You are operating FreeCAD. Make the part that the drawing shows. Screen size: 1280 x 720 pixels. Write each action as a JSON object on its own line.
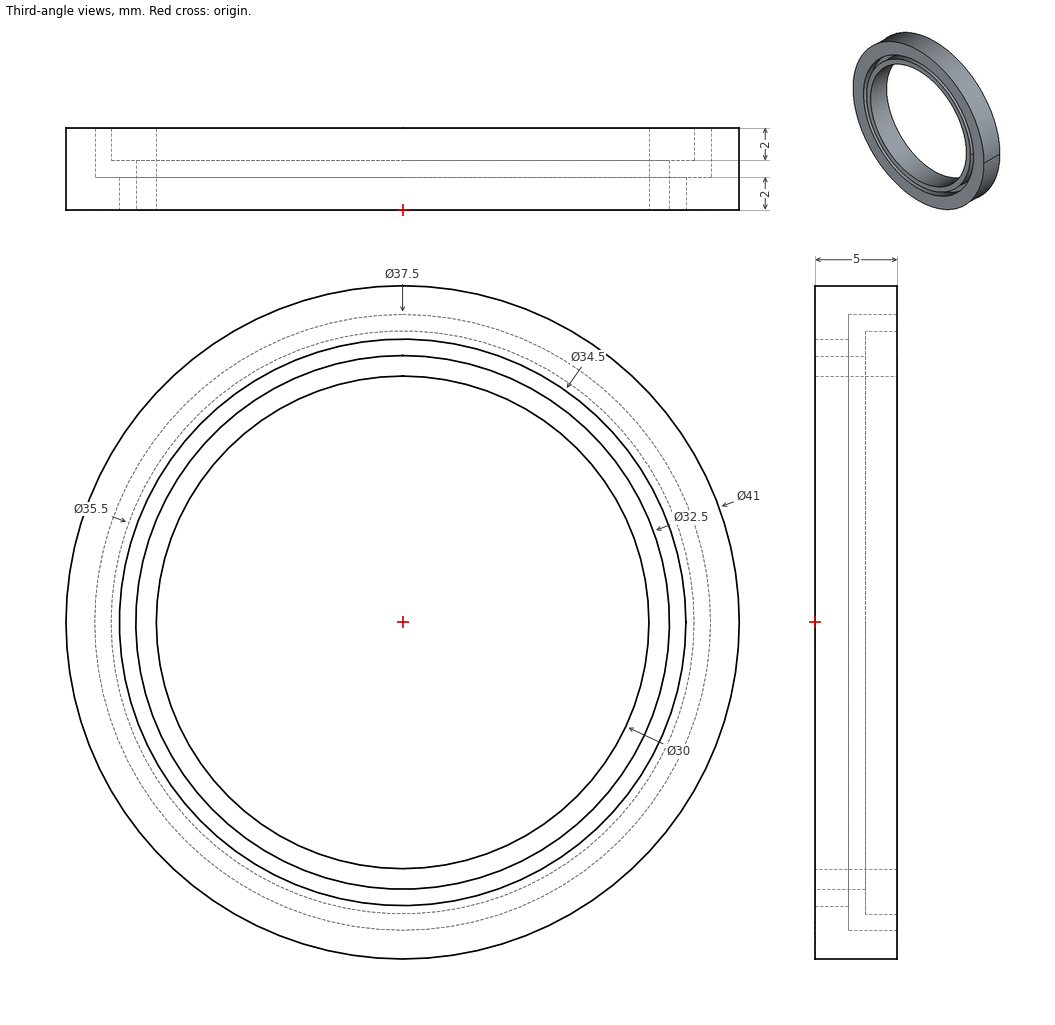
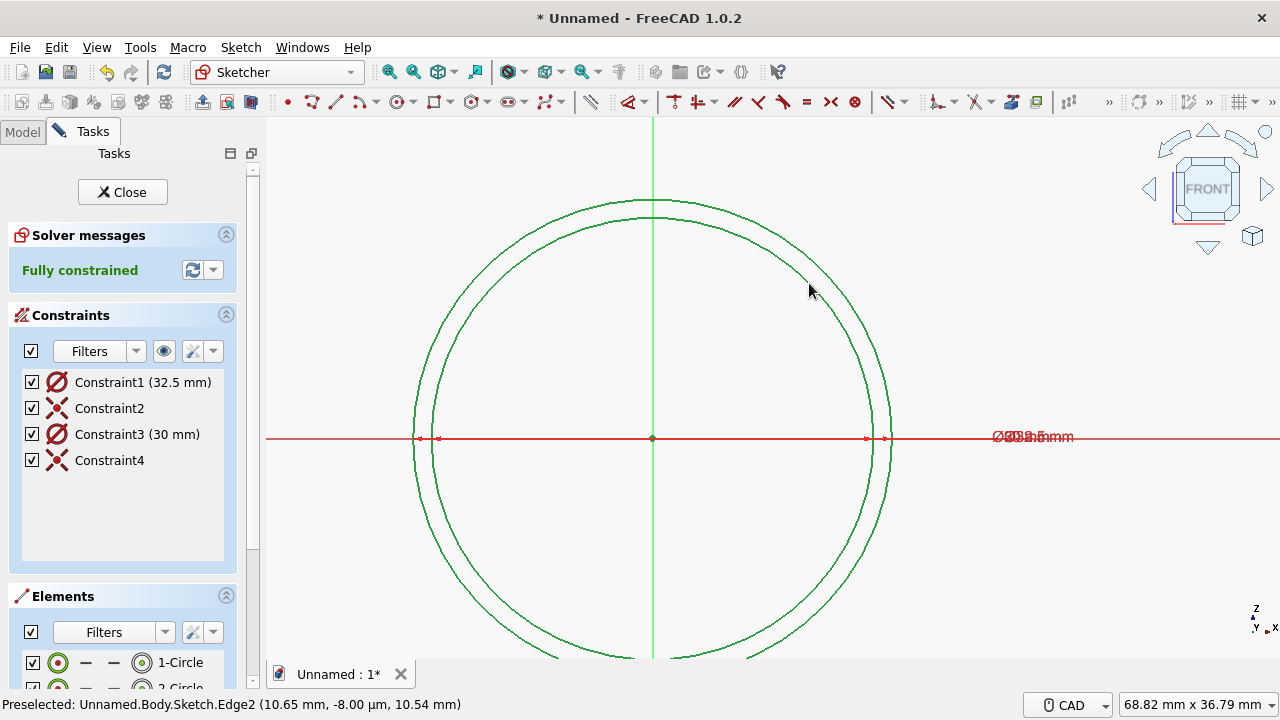
{"action": "left_click", "coordinate": [123, 192]}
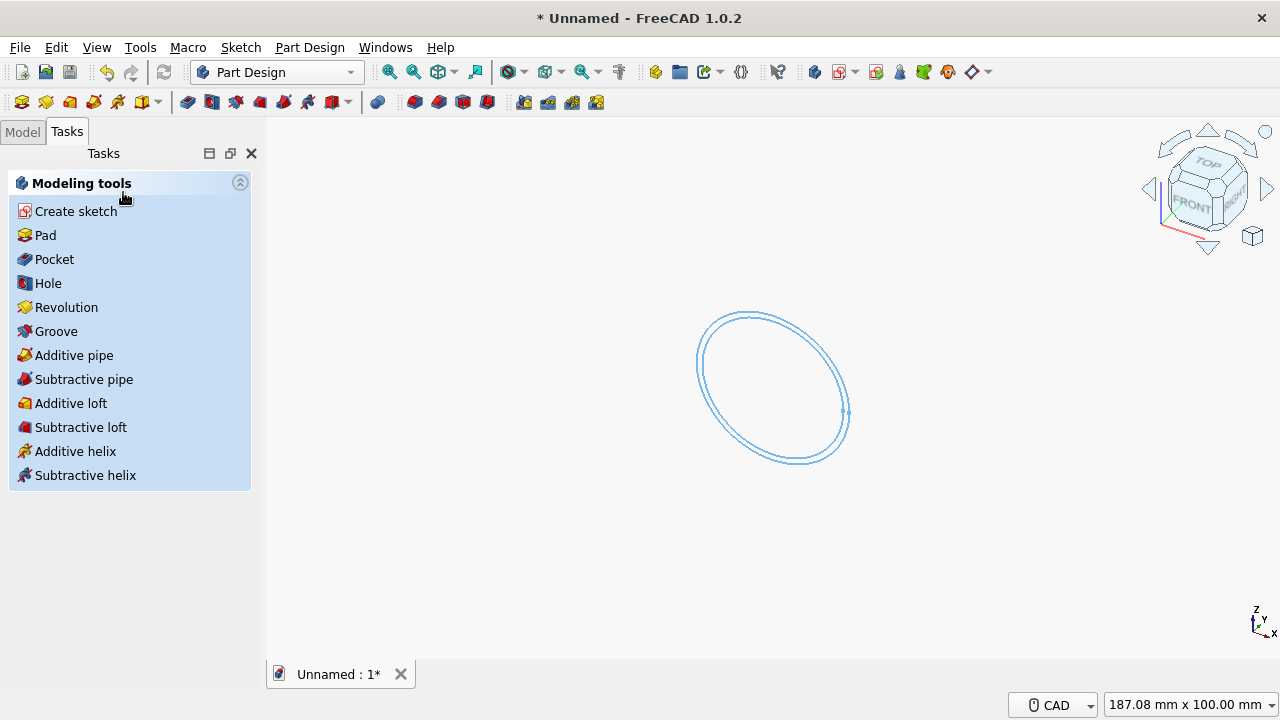
{"action": "left_click", "coordinate": [22, 102]}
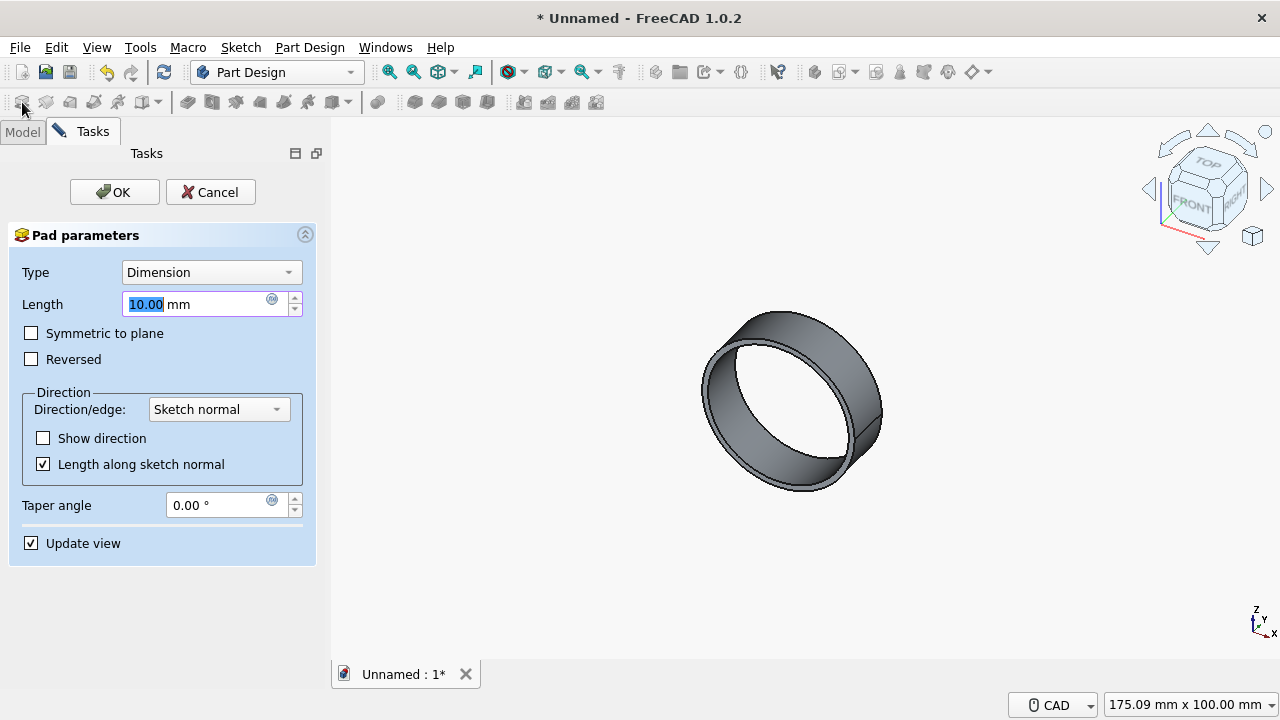
{"action": "type", "text": "5"}
{"action": "key", "text": "Tab"}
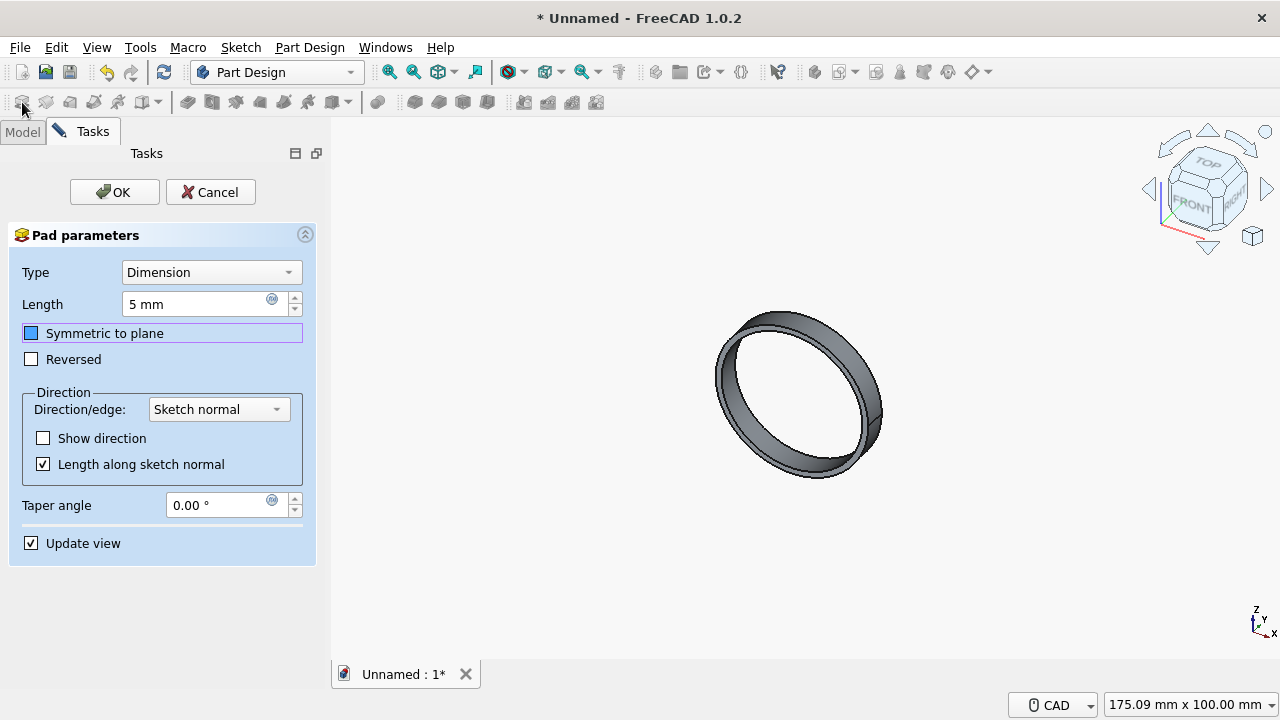
{"action": "left_click", "coordinate": [30, 359]}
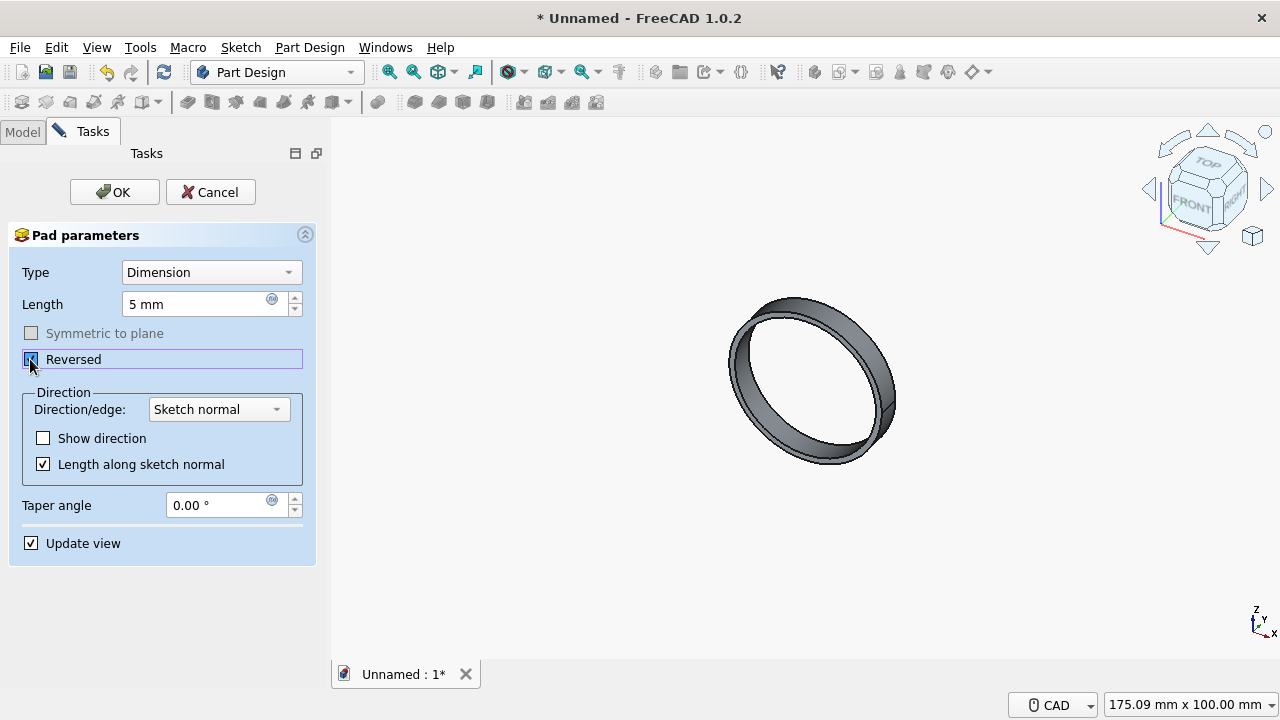
{"action": "left_click", "coordinate": [115, 192]}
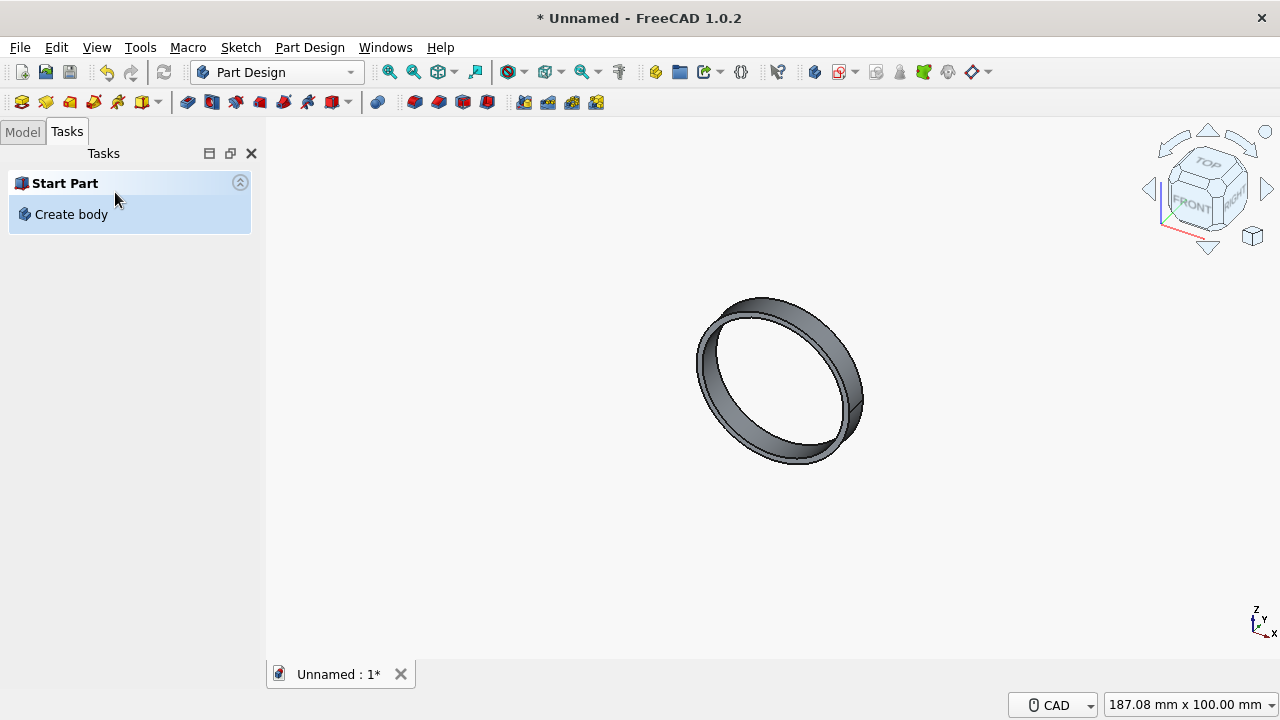
{"action": "key", "text": "v f"}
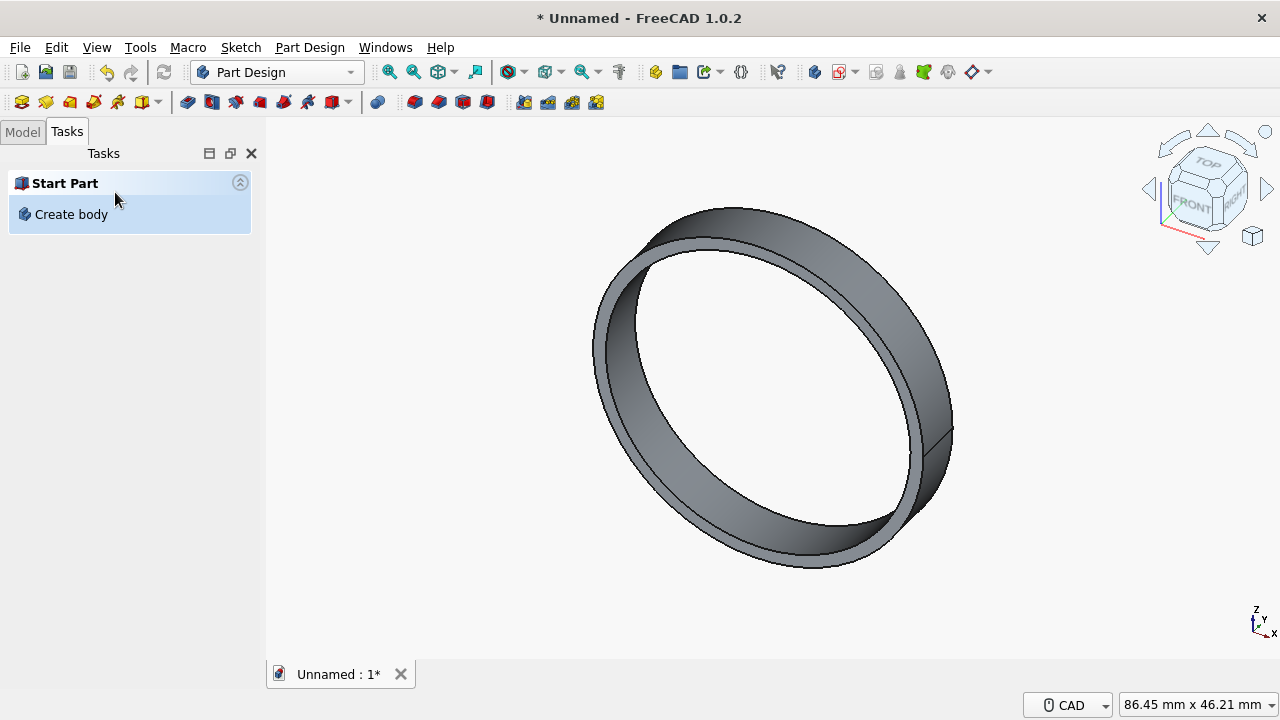
{"action": "left_click", "coordinate": [23, 131]}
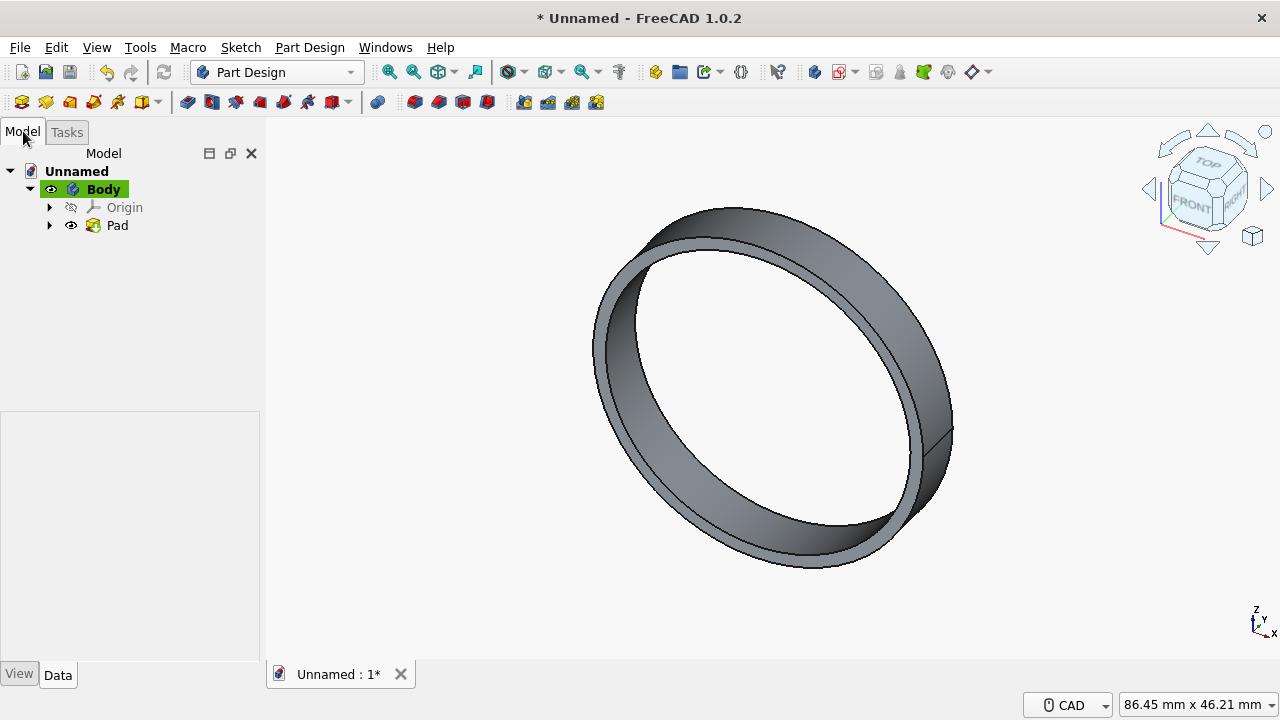
{"action": "left_click", "coordinate": [50, 207]}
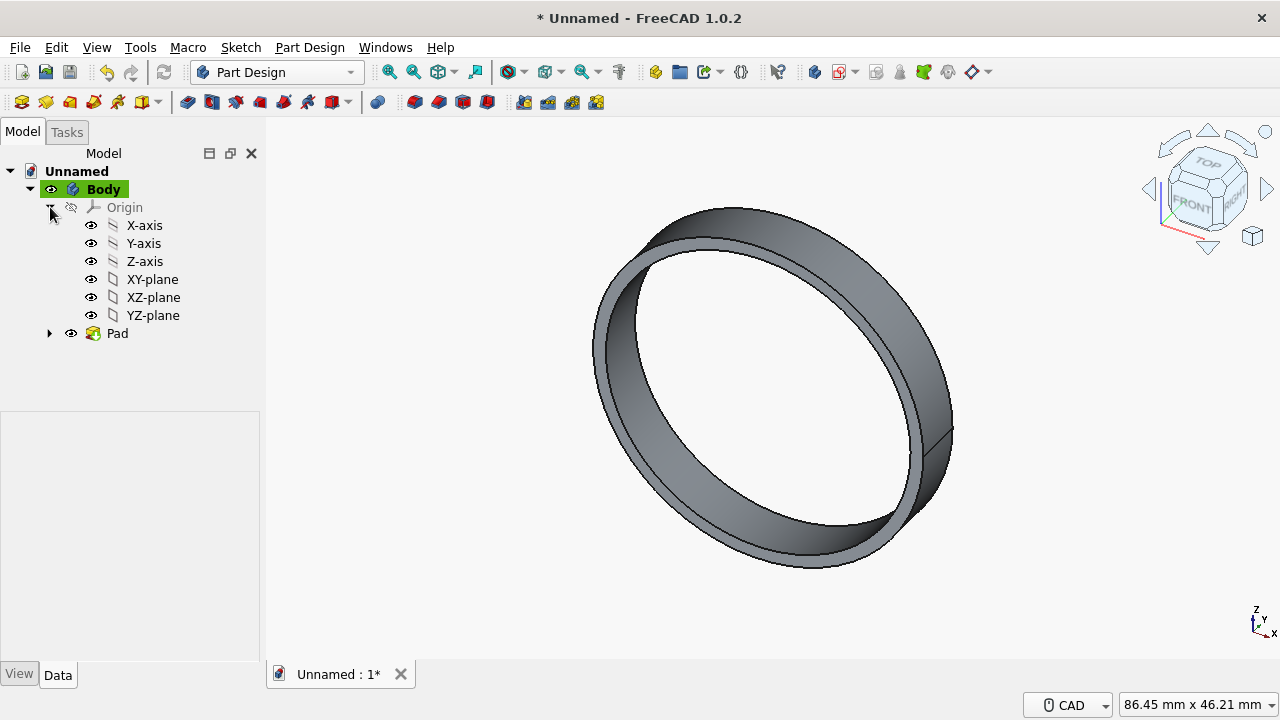
{"action": "left_click", "coordinate": [136, 297]}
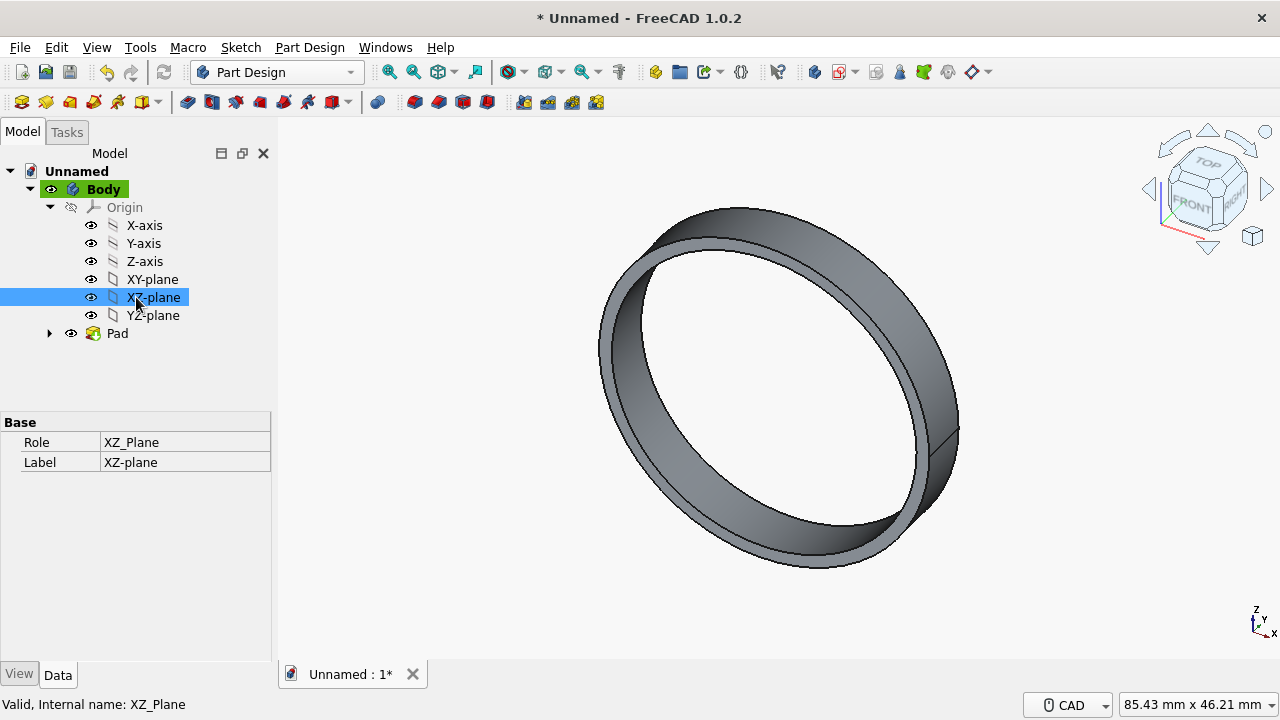
{"action": "left_click", "coordinate": [972, 72]}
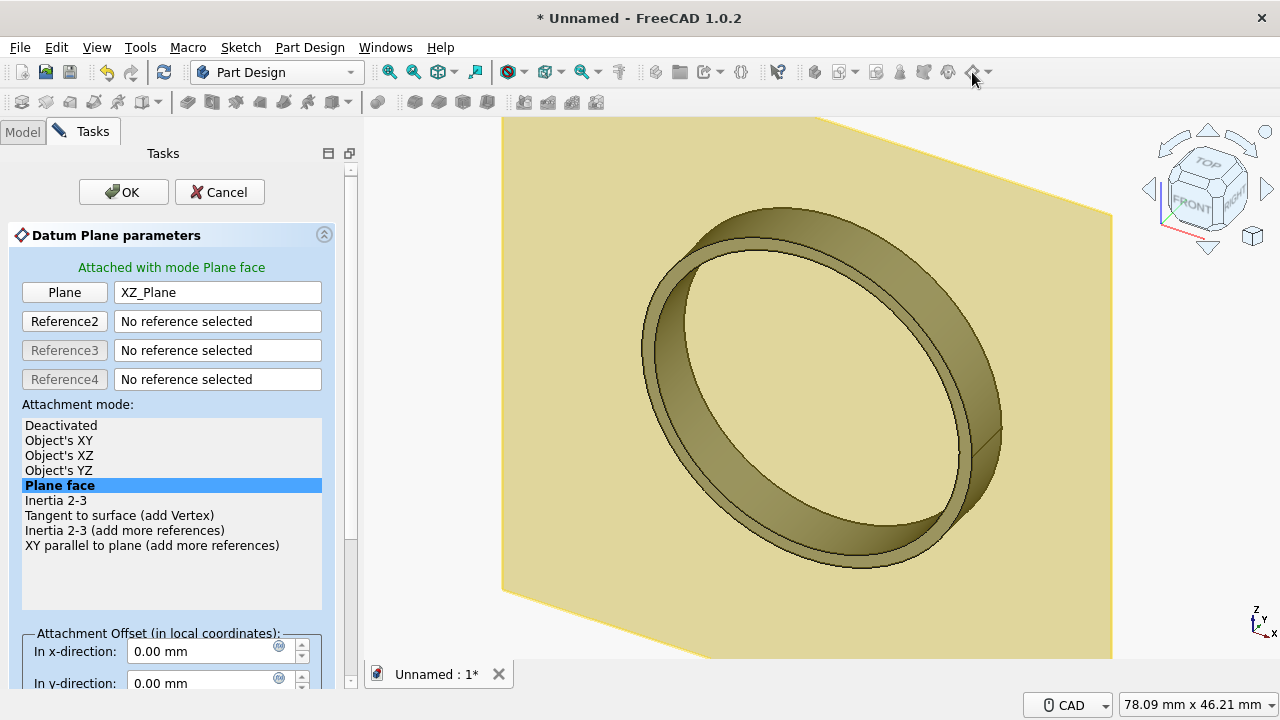
{"action": "scroll", "coordinate": [351, 426], "scroll_direction": "down", "scroll_amount": 2}